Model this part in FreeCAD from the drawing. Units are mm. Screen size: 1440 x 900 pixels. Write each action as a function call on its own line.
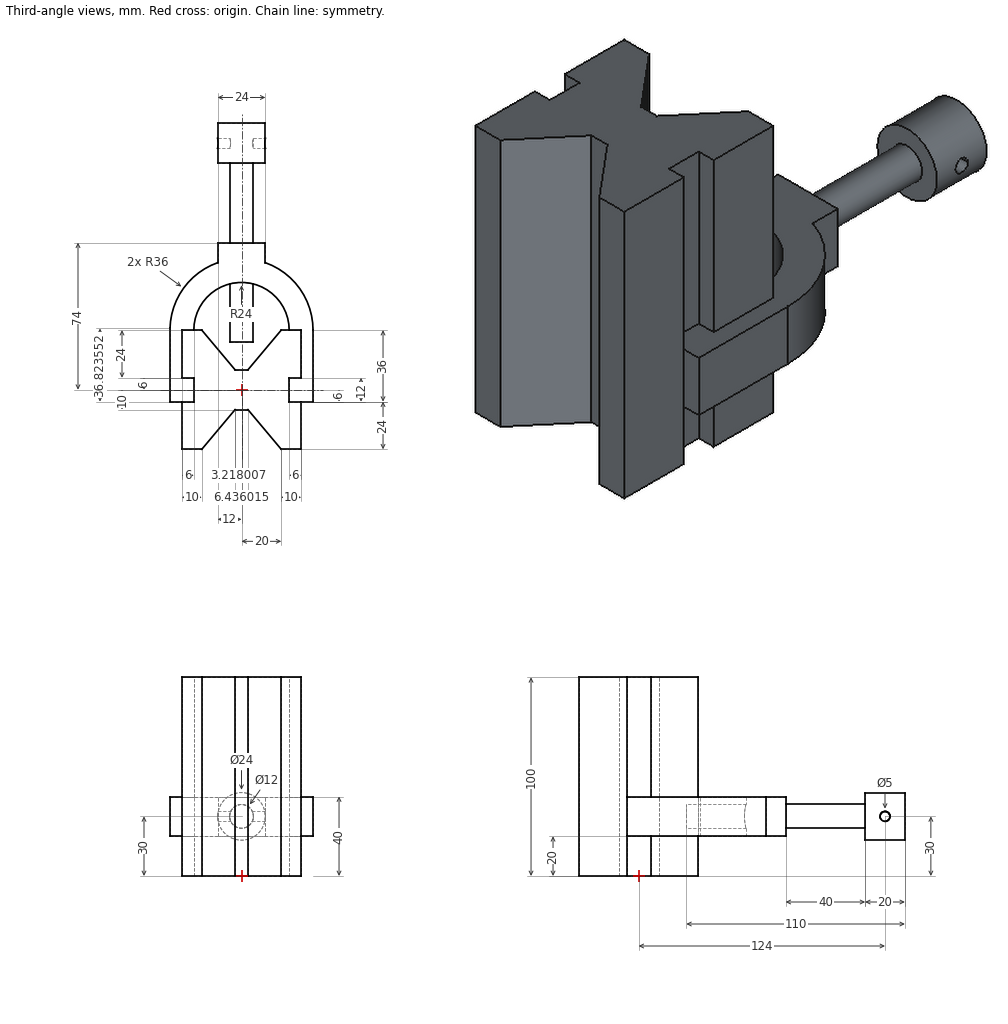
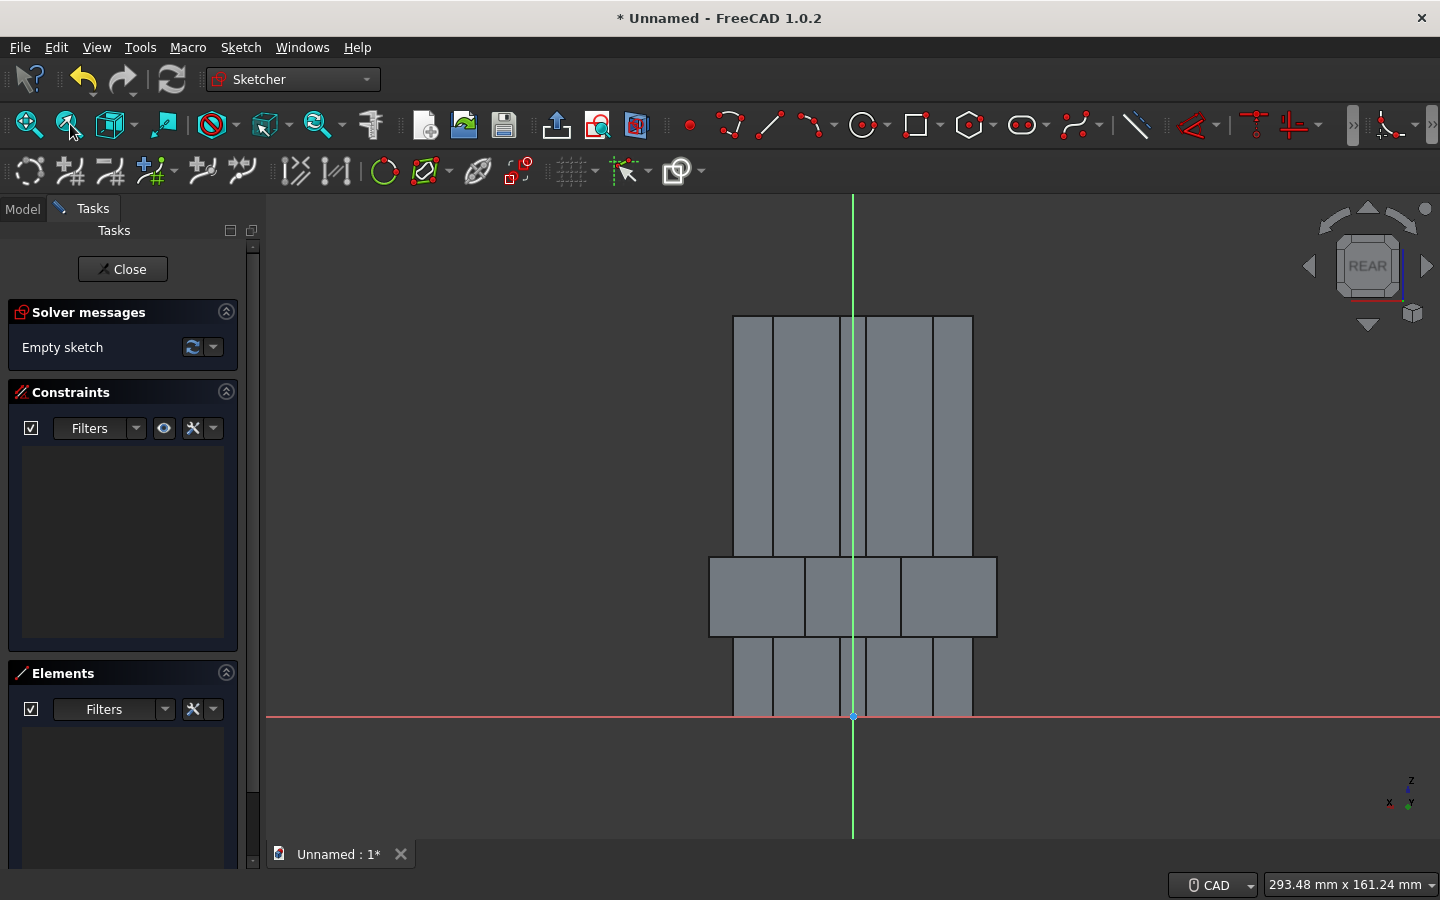
scroll(862, 606, up, 11)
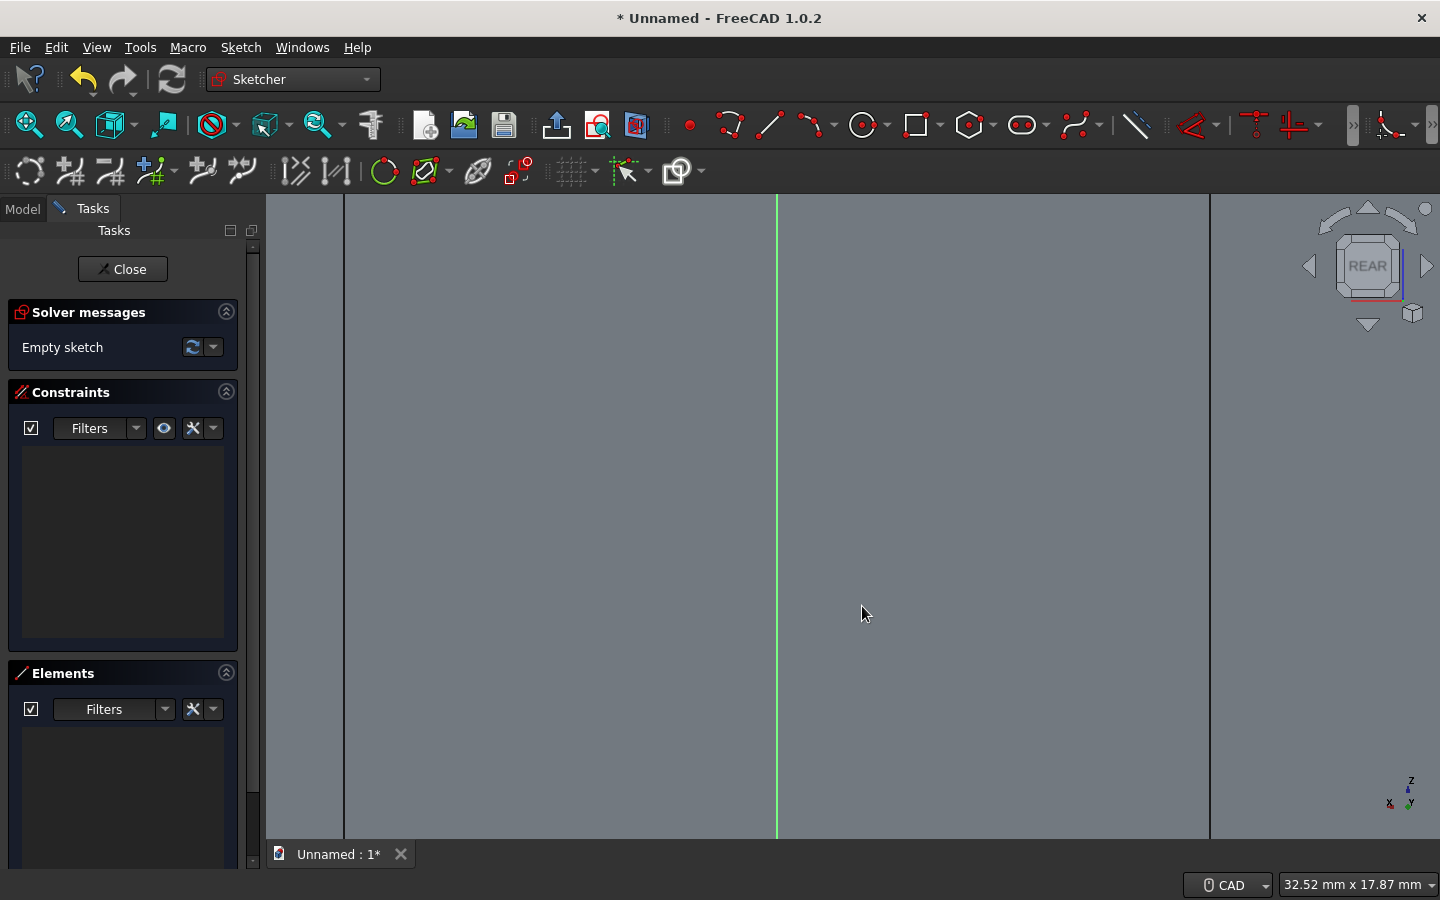
key(g)
key(c)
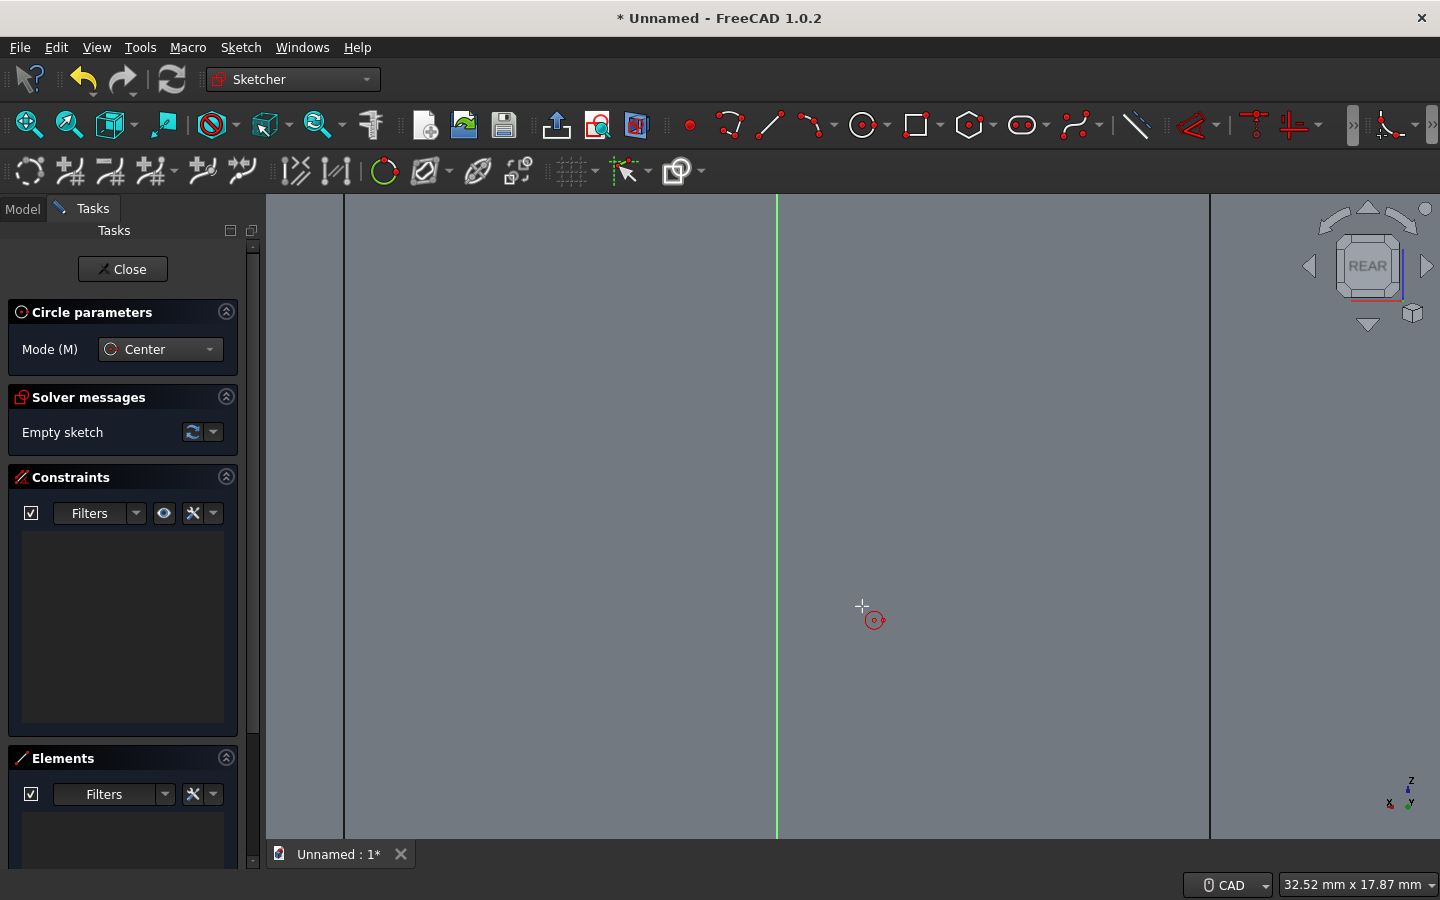
click(777, 515)
move(930, 362)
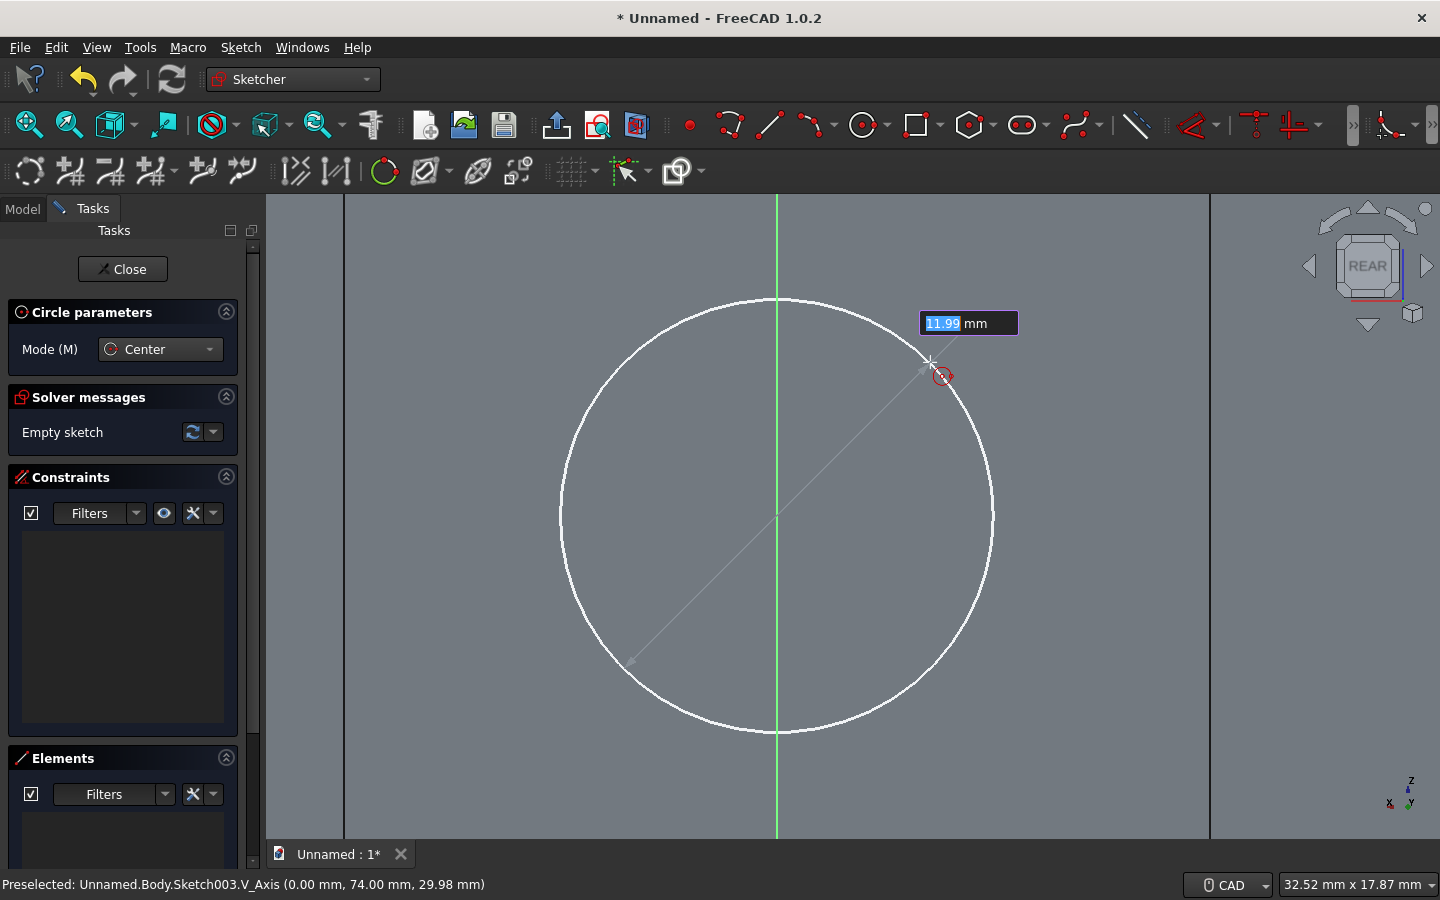
text(12)
key(Return)
key(Escape)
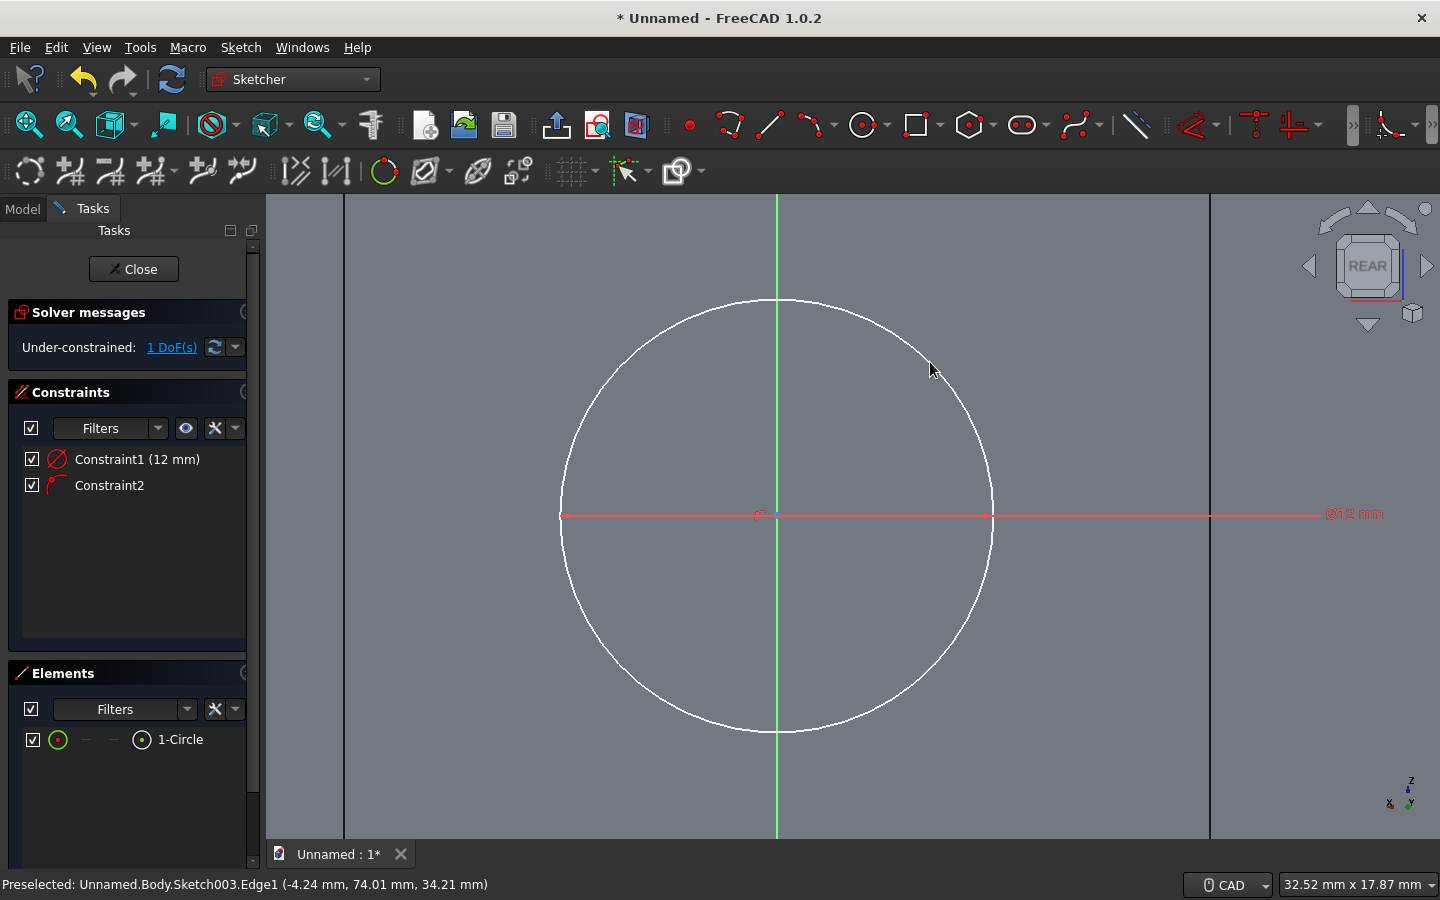
click(1192, 126)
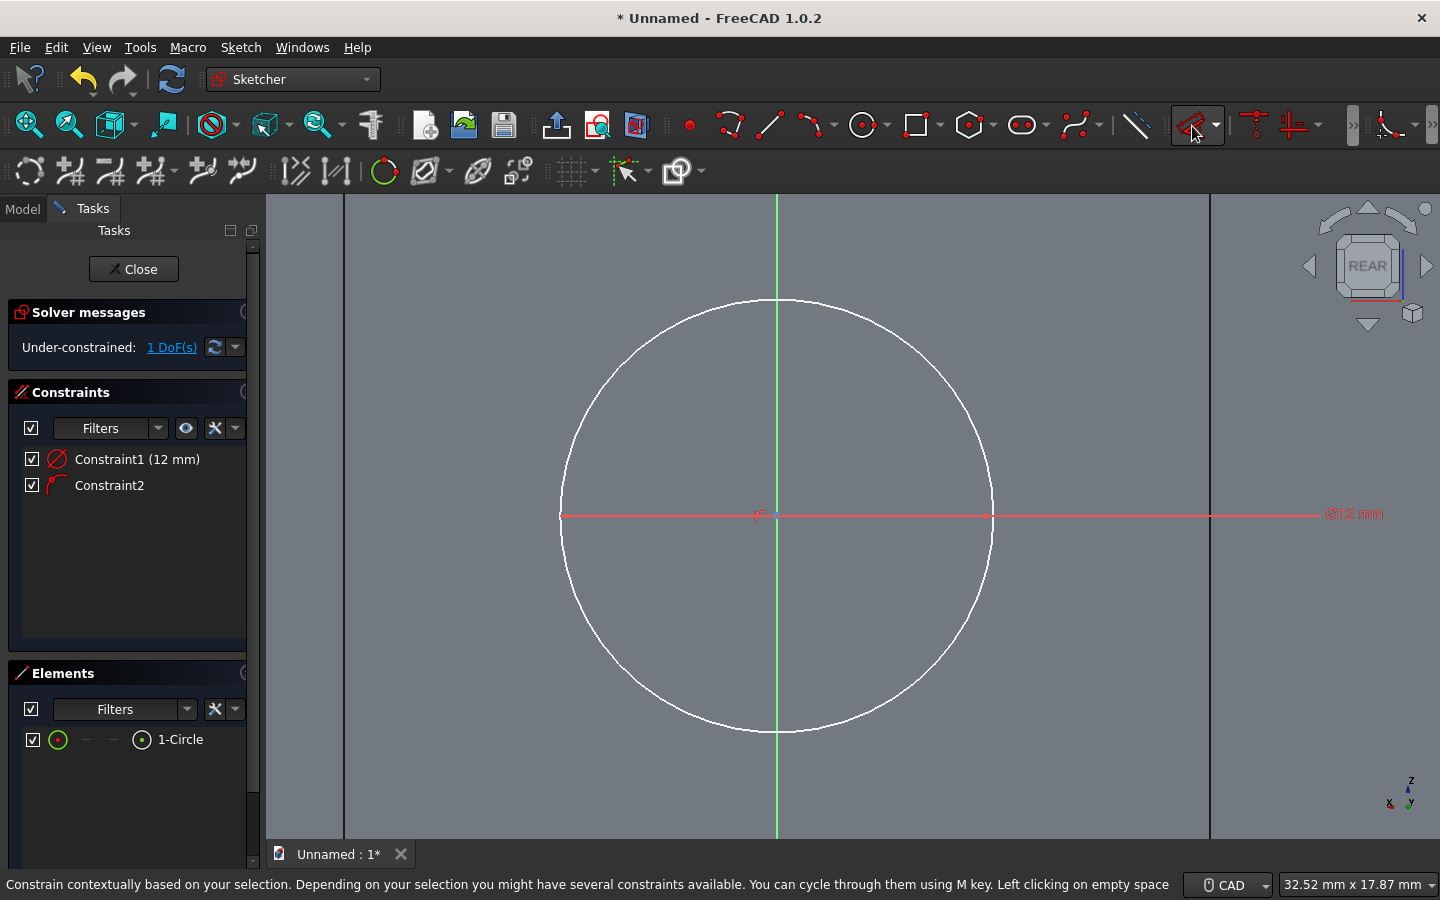
click(777, 516)
click(811, 664)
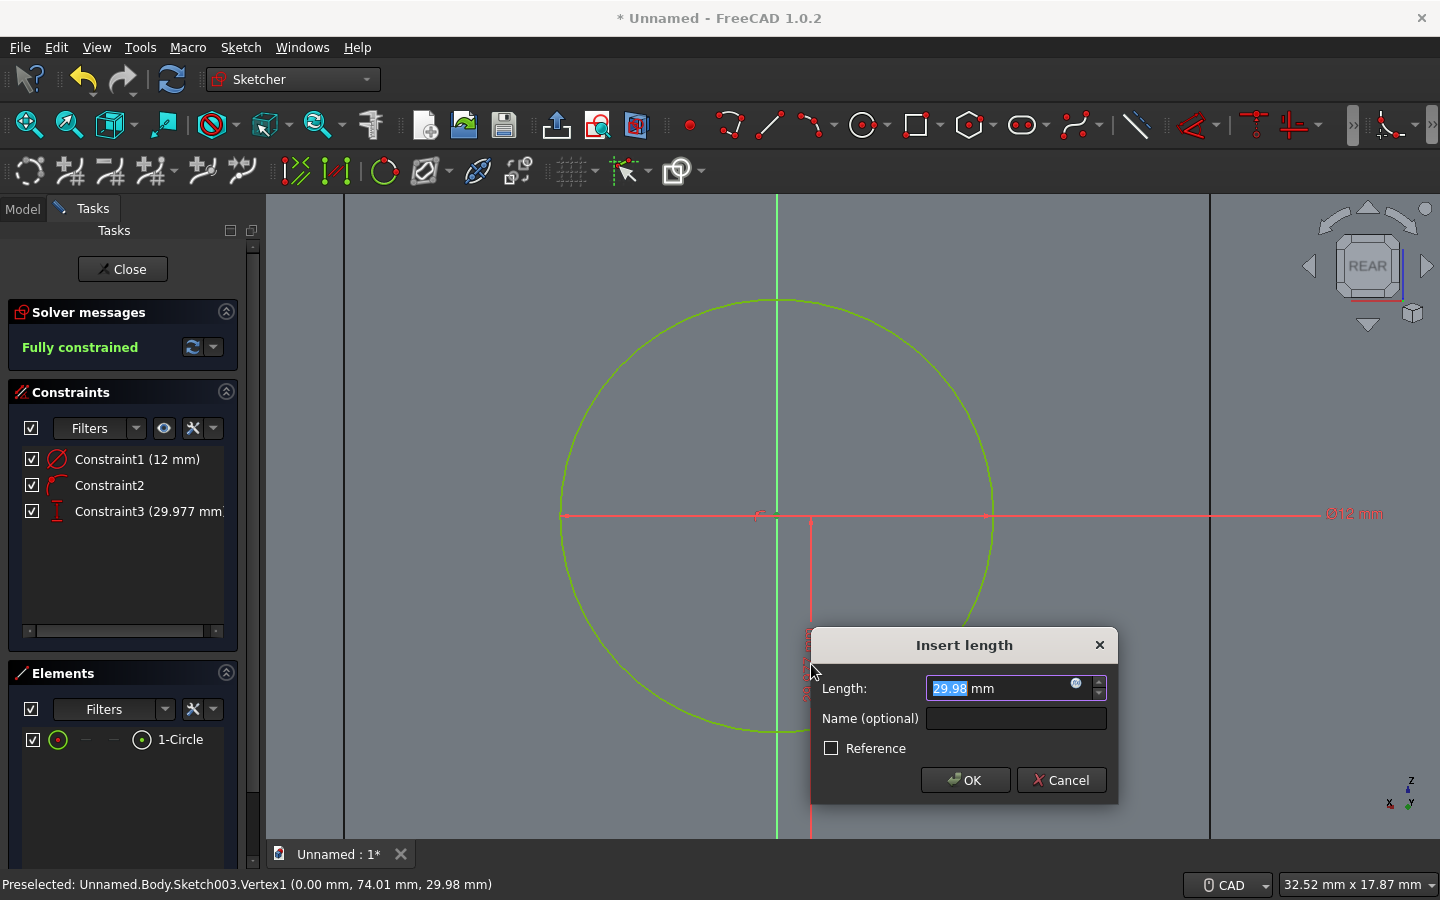
text(30)
key(Return)
key(Escape)